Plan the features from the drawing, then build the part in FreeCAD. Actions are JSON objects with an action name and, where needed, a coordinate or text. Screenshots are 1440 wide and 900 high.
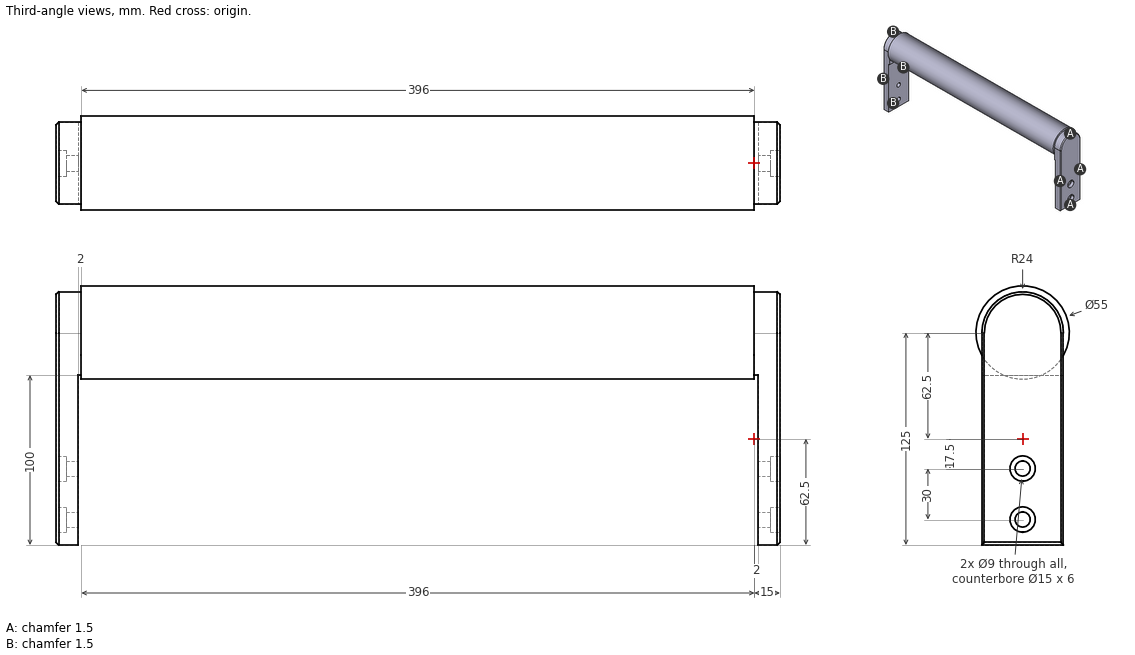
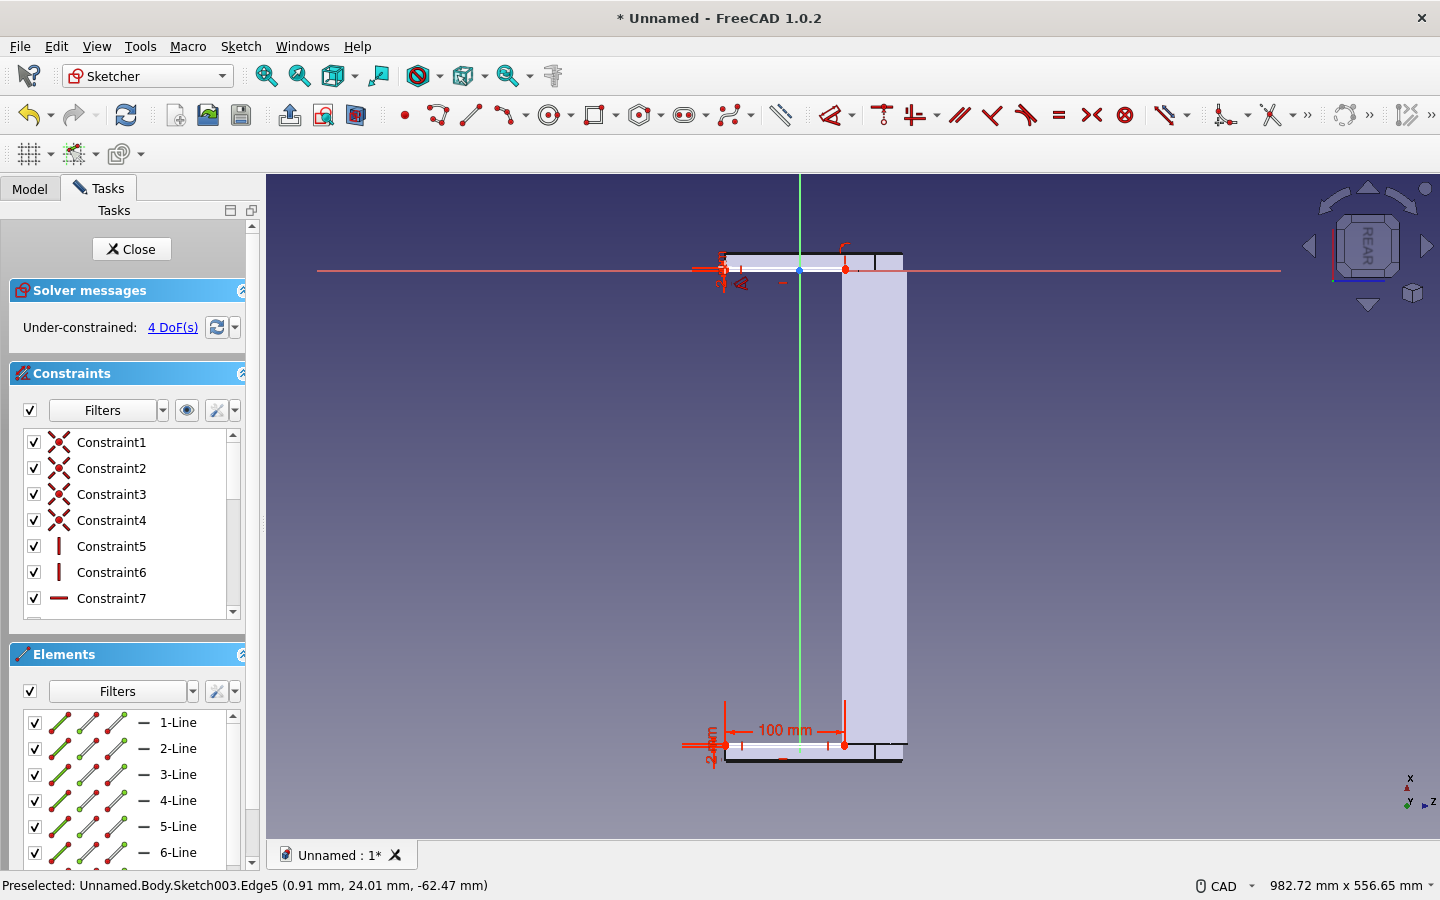
{"action": "scroll", "coordinate": [749, 271], "scroll_direction": "up", "scroll_amount": 9}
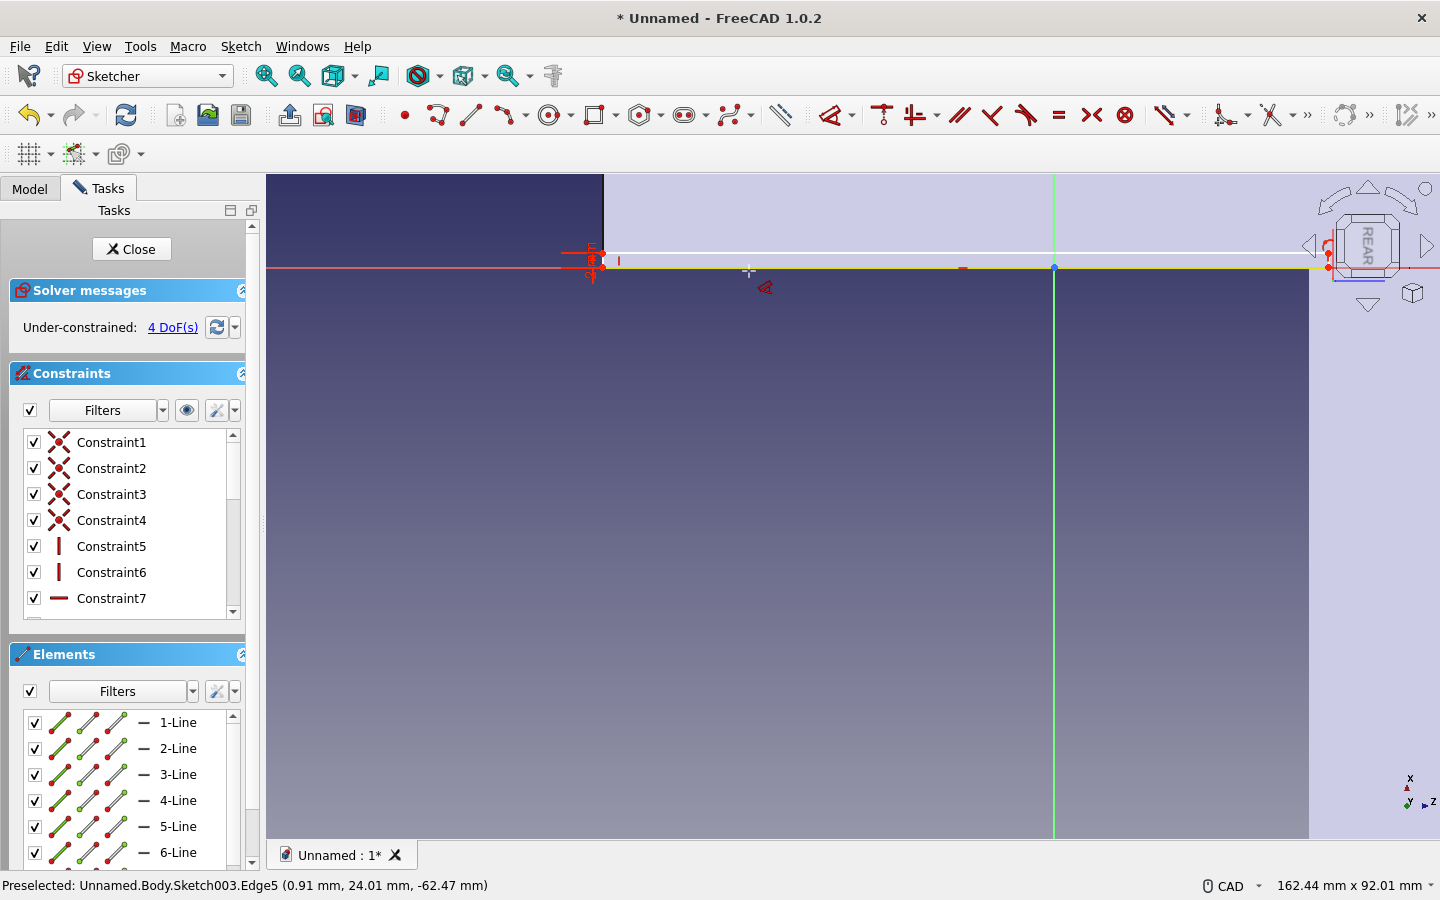
{"action": "left_click", "coordinate": [748, 268]}
{"action": "left_click", "coordinate": [939, 234]}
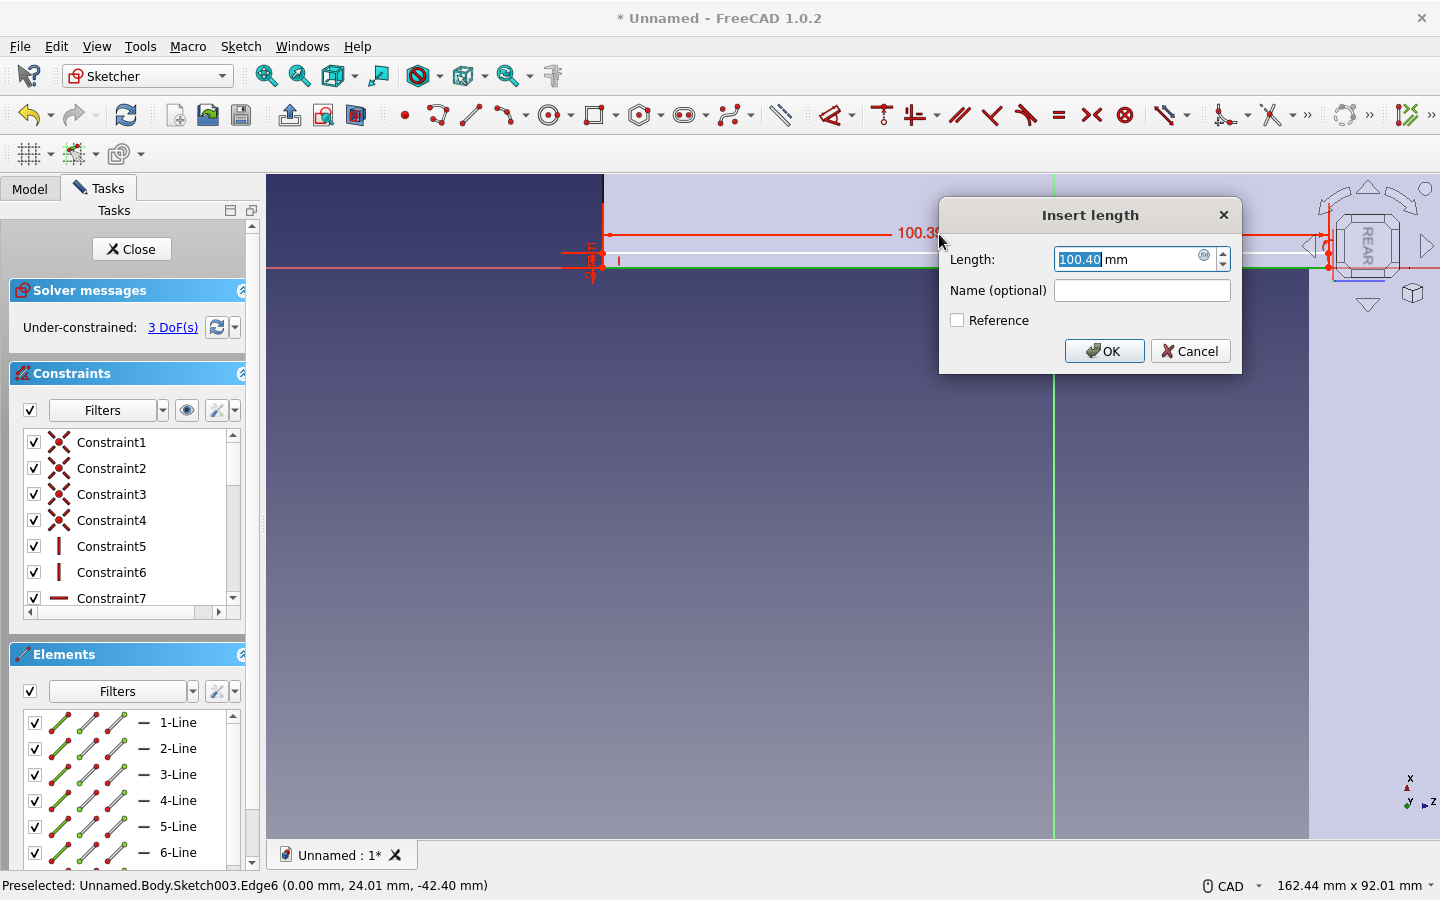
{"action": "type", "text": "100"}
{"action": "key", "text": "Return"}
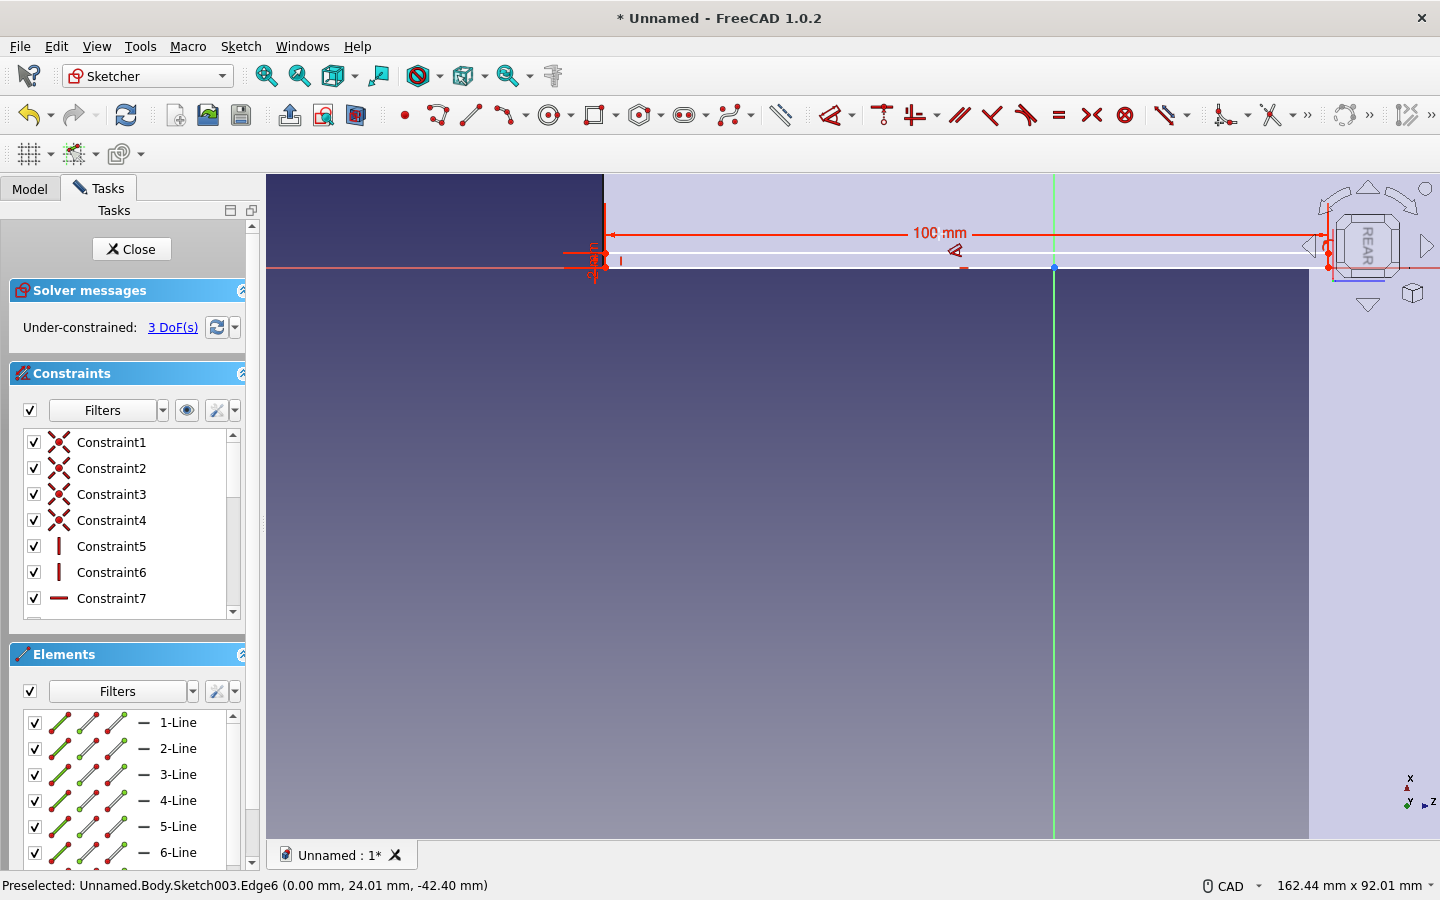
{"action": "scroll", "coordinate": [756, 320], "scroll_direction": "down", "scroll_amount": 10}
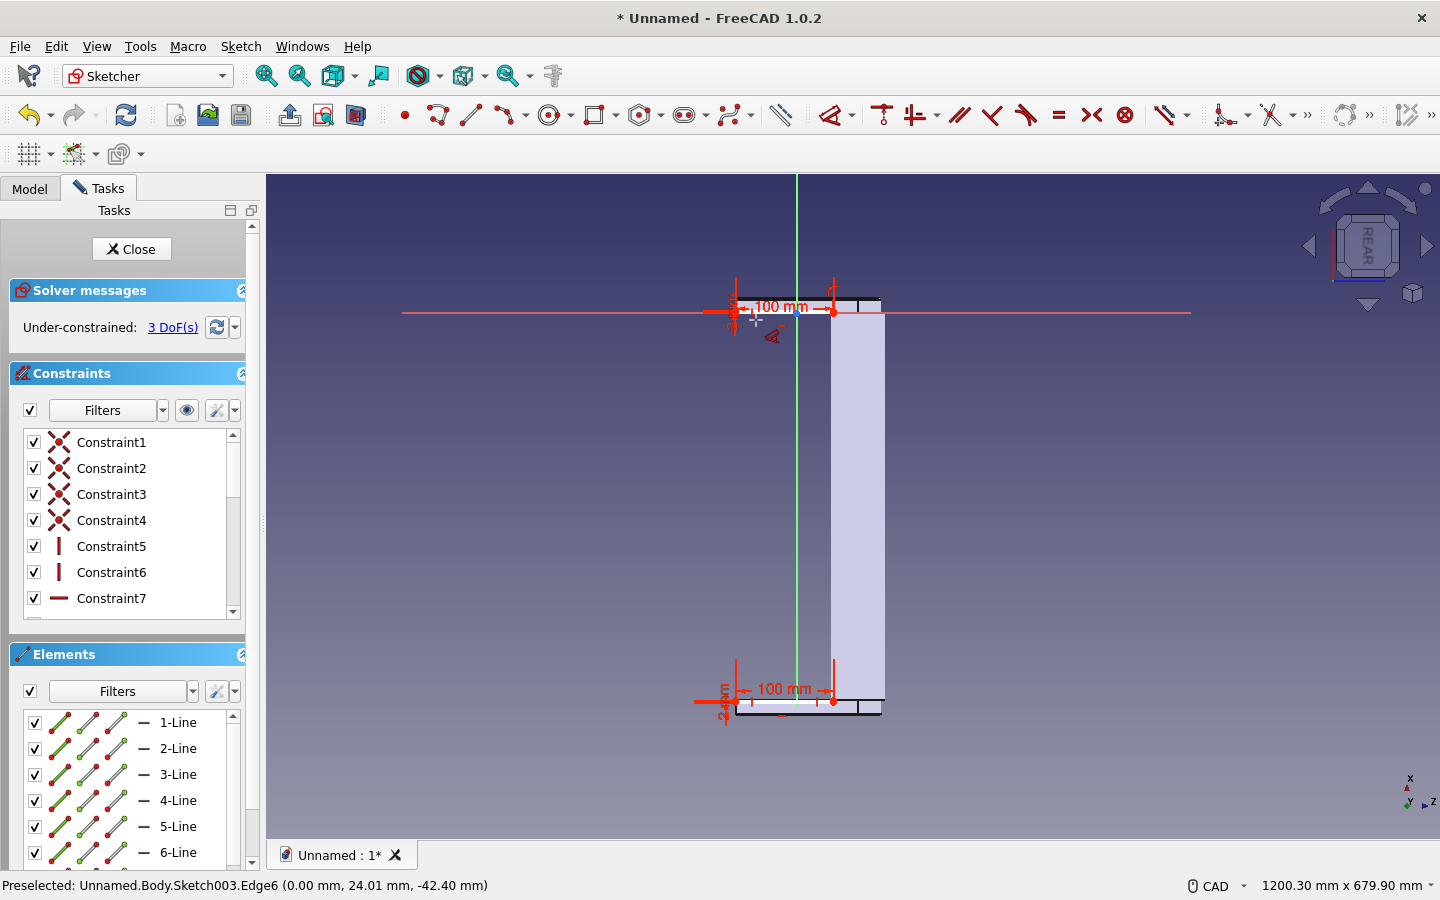
{"action": "scroll", "coordinate": [736, 701], "scroll_direction": "up", "scroll_amount": 10}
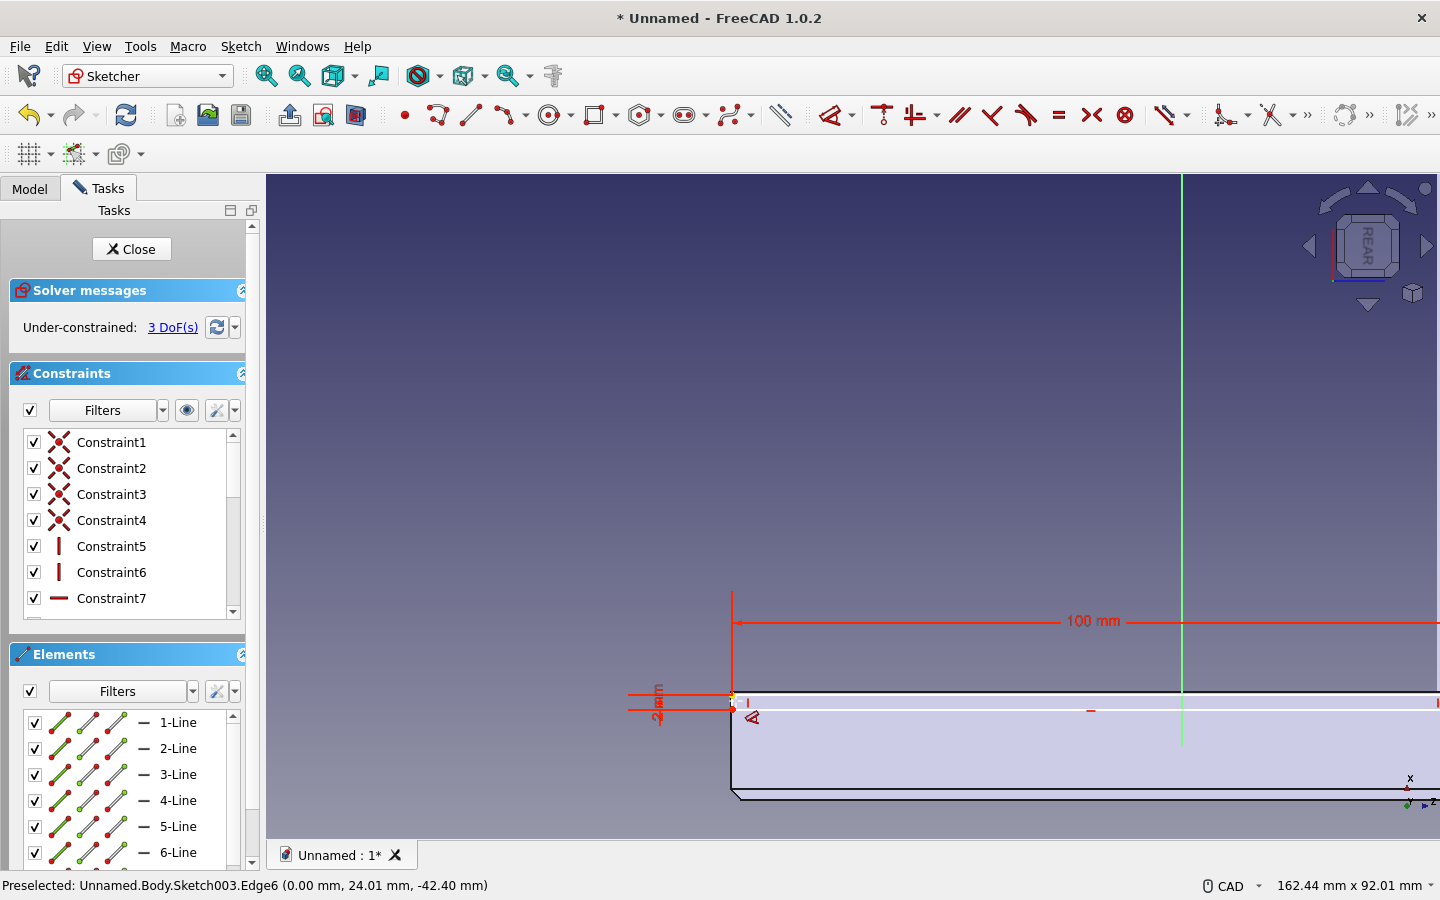
{"action": "left_click", "coordinate": [732, 695]}
{"action": "left_click", "coordinate": [698, 449]}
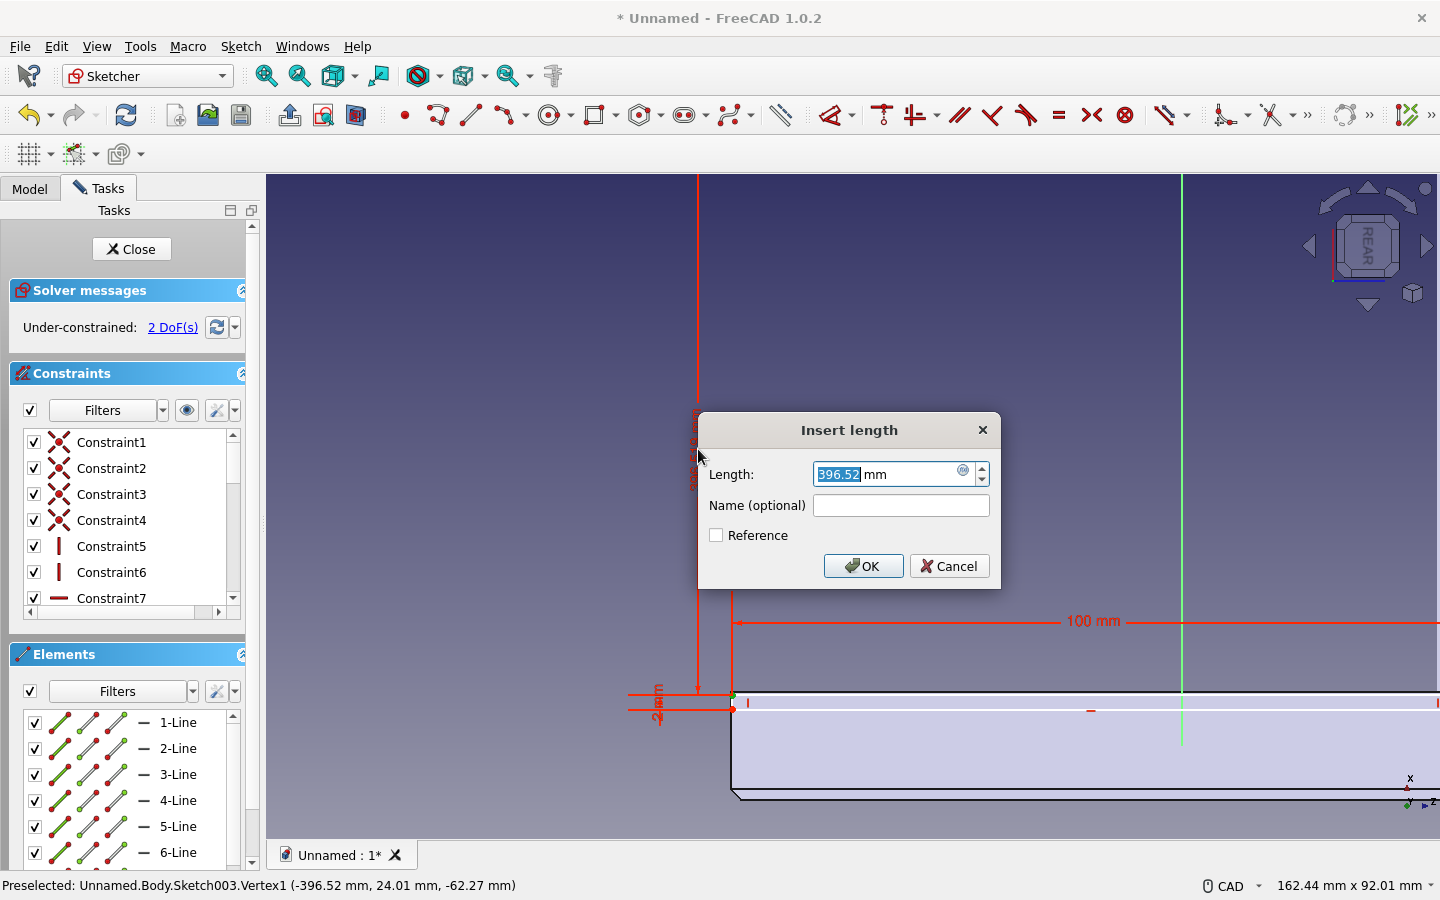
{"action": "type", "text": "396"}
{"action": "key", "text": "Return"}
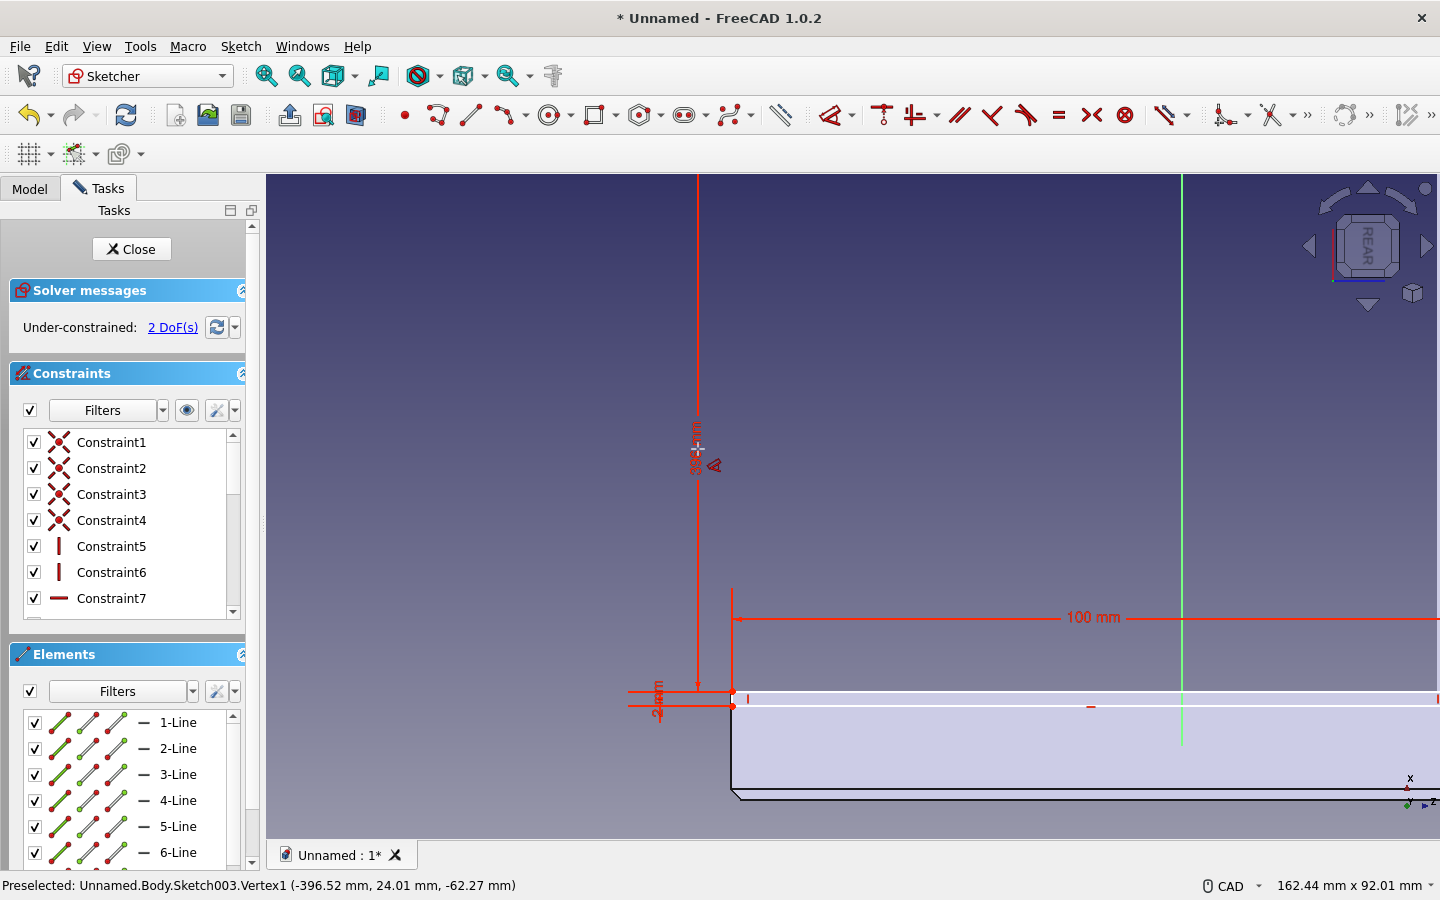
{"action": "left_click", "coordinate": [732, 692]}
{"action": "left_click", "coordinate": [957, 726]}